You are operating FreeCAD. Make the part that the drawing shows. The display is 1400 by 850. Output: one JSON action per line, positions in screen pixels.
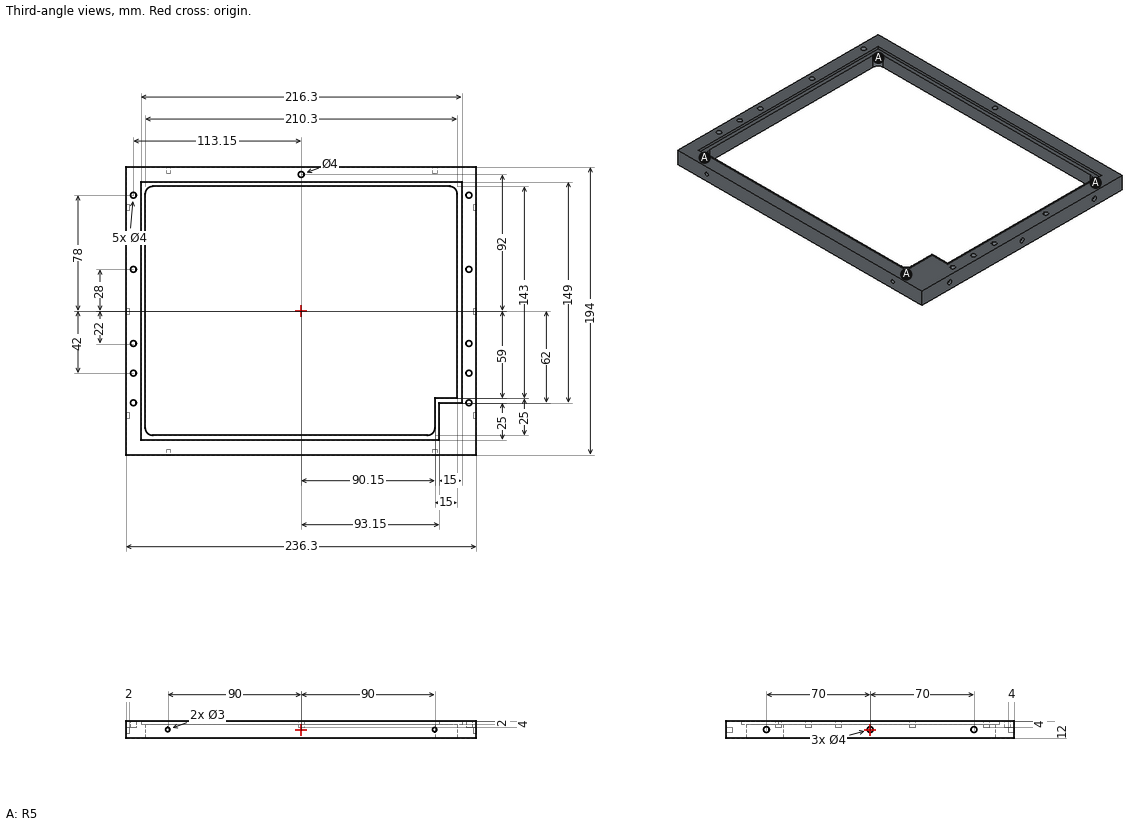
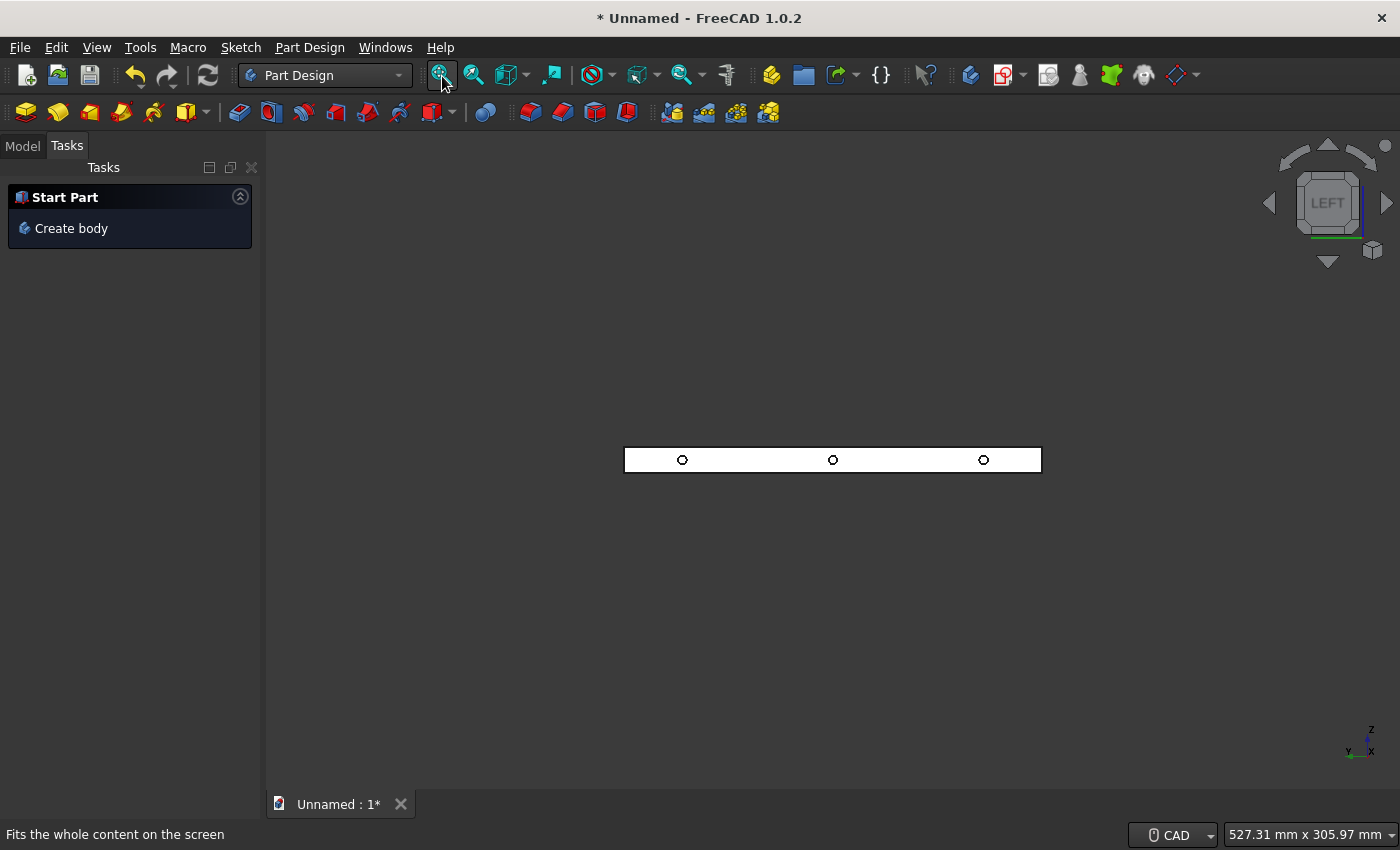
{"action": "left_click", "coordinate": [23, 145]}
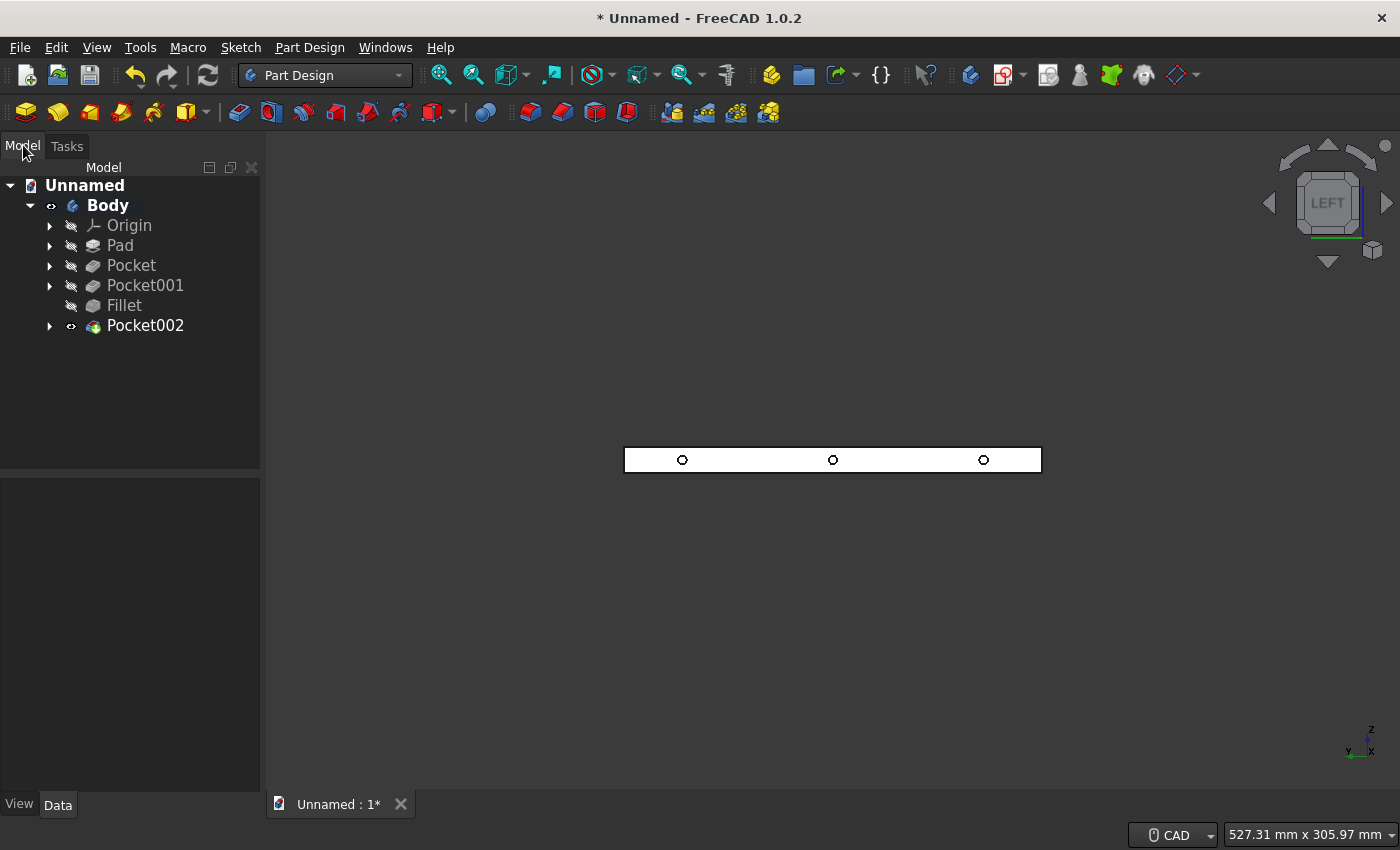
{"action": "left_click", "coordinate": [116, 326]}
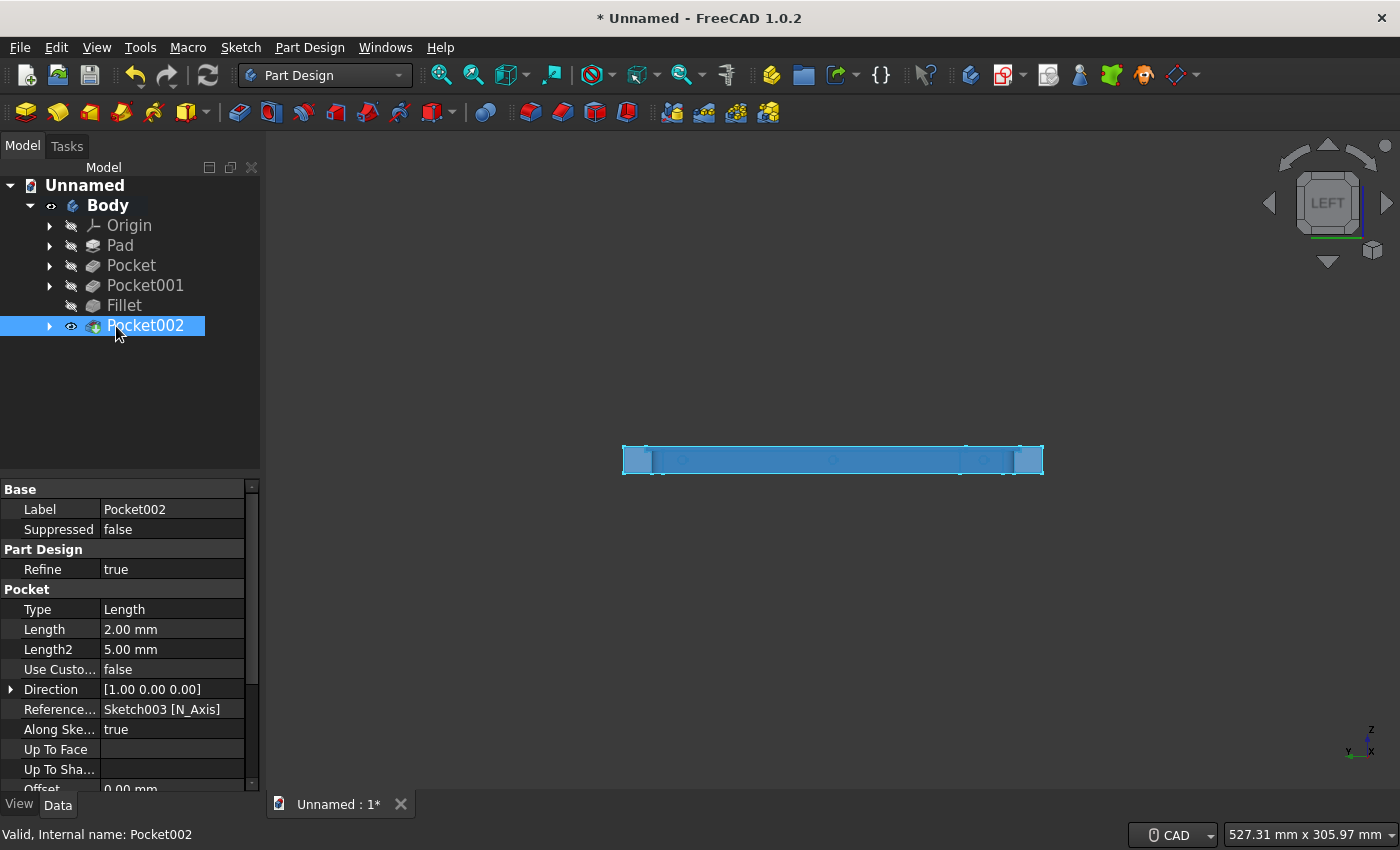
{"action": "left_click", "coordinate": [672, 112]}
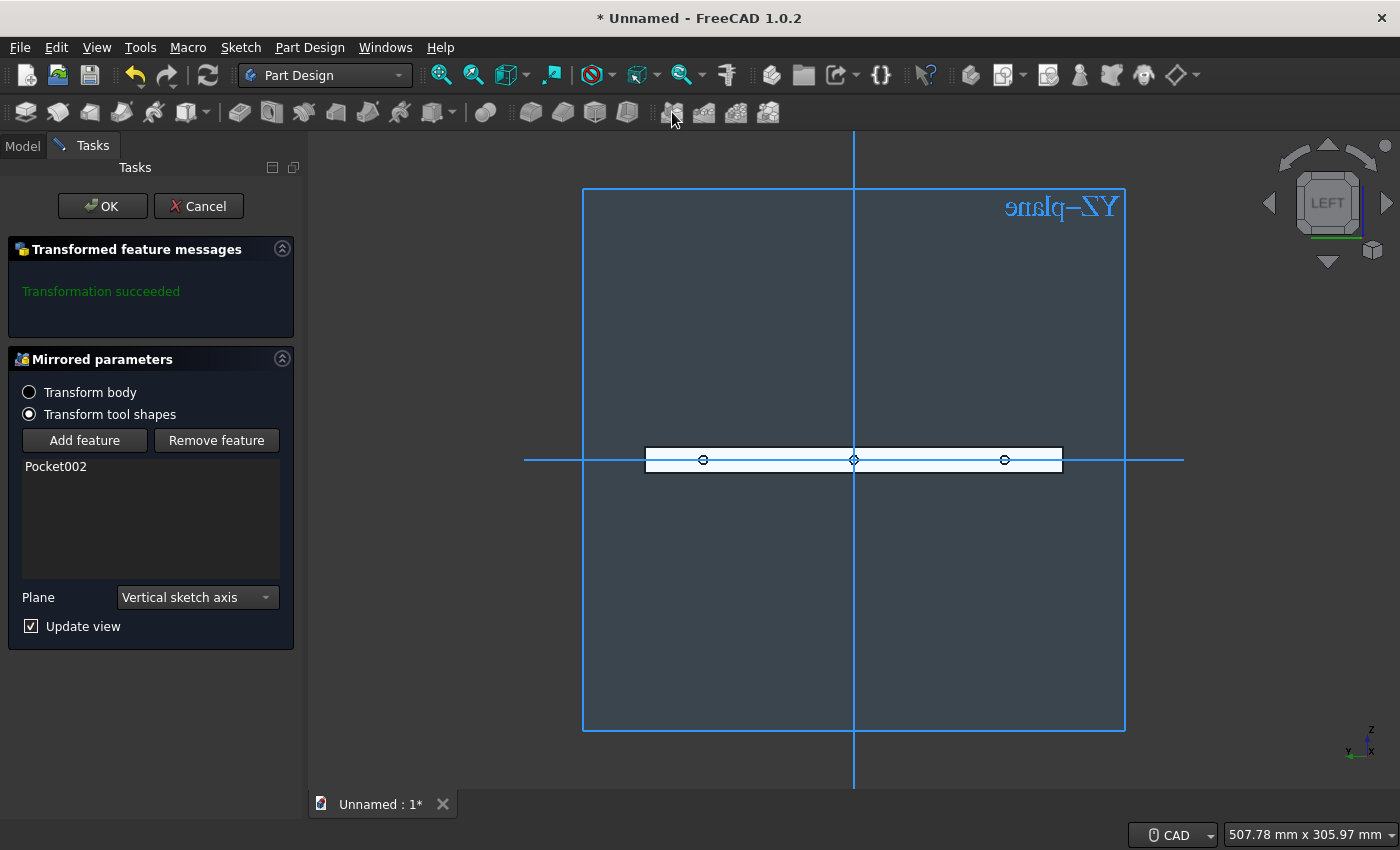
{"action": "left_click", "coordinate": [198, 598]}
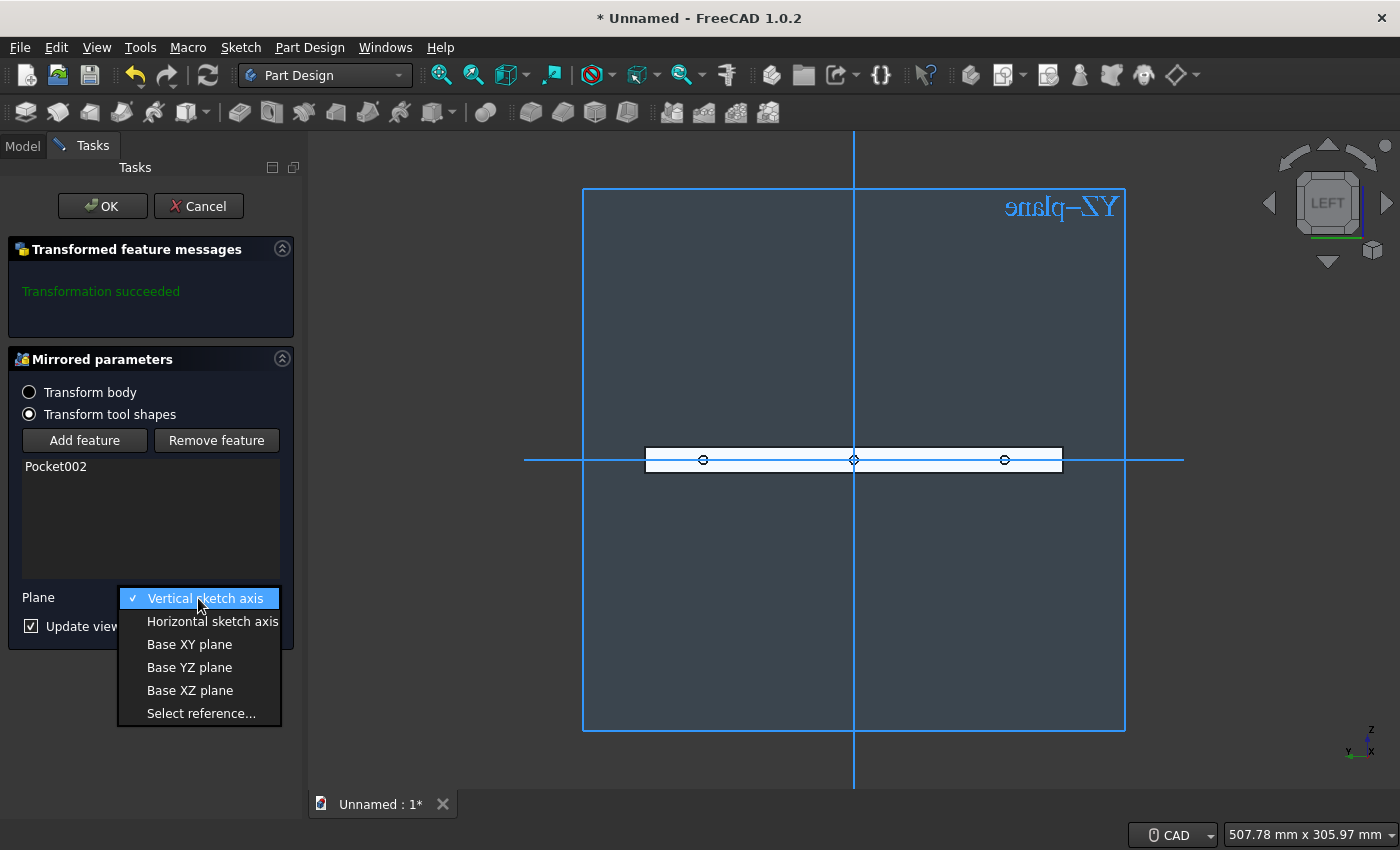
{"action": "left_click", "coordinate": [198, 668]}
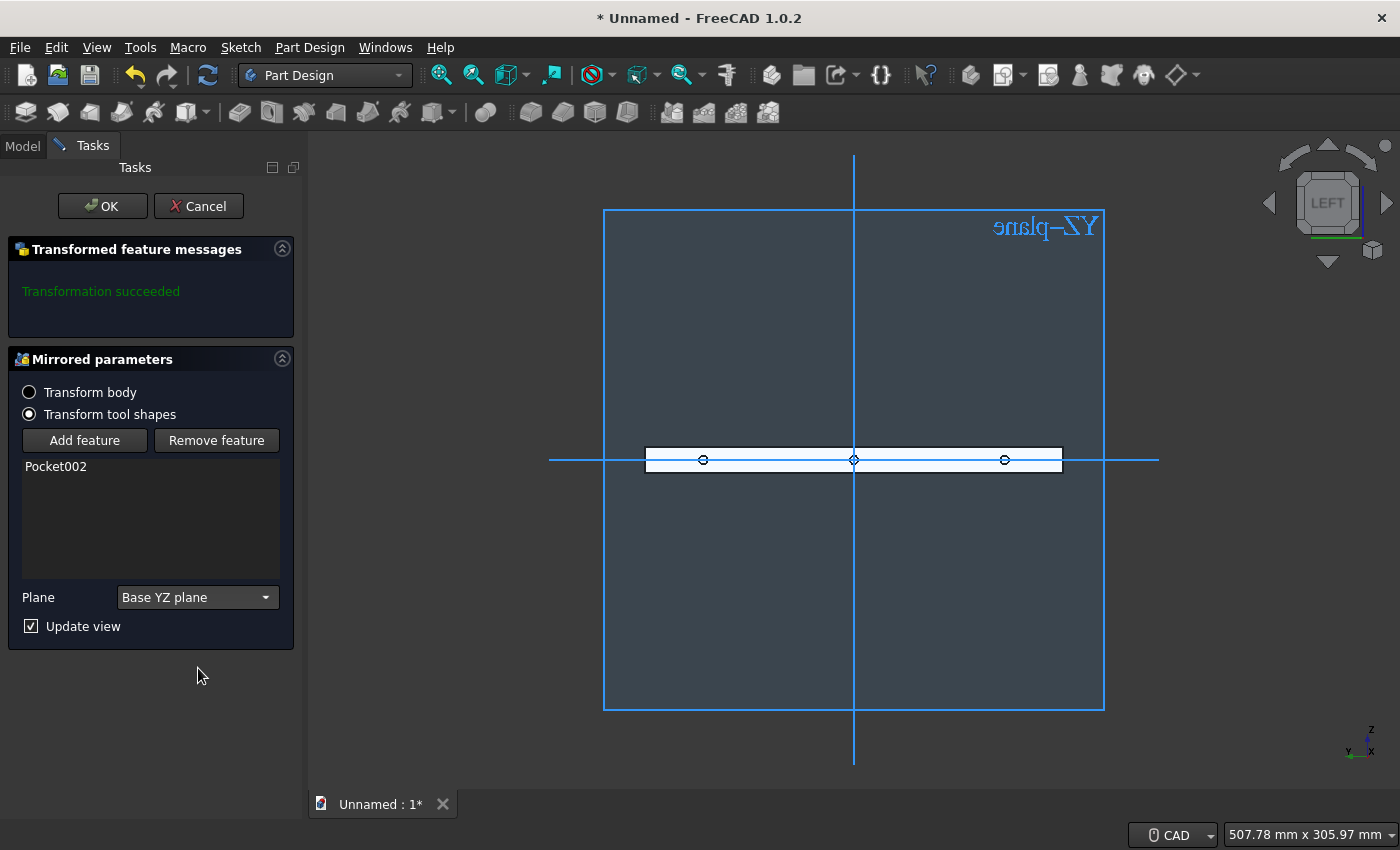
{"action": "left_click", "coordinate": [103, 206]}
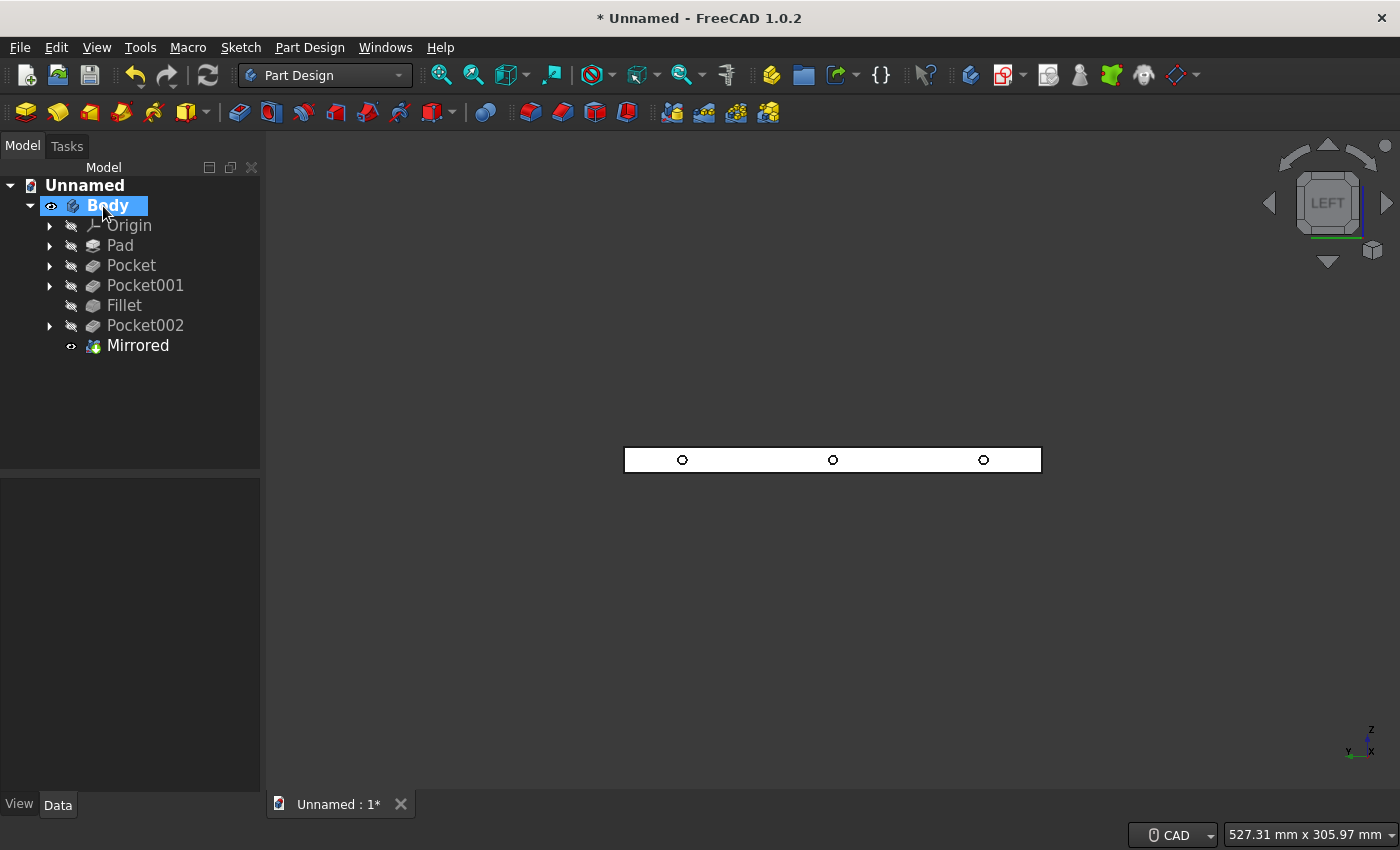
{"action": "left_click", "coordinate": [442, 76]}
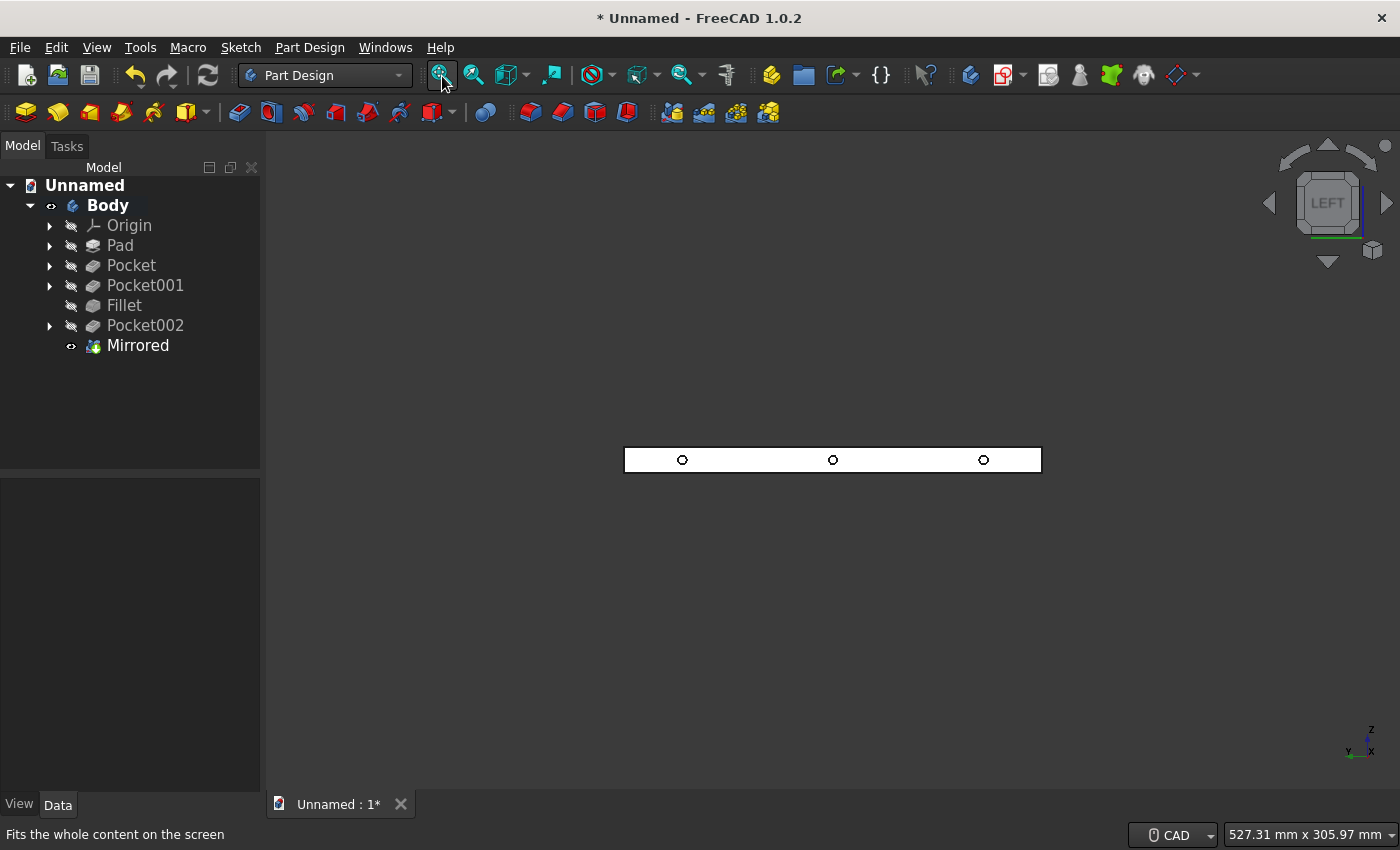
{"action": "key", "text": "4"}